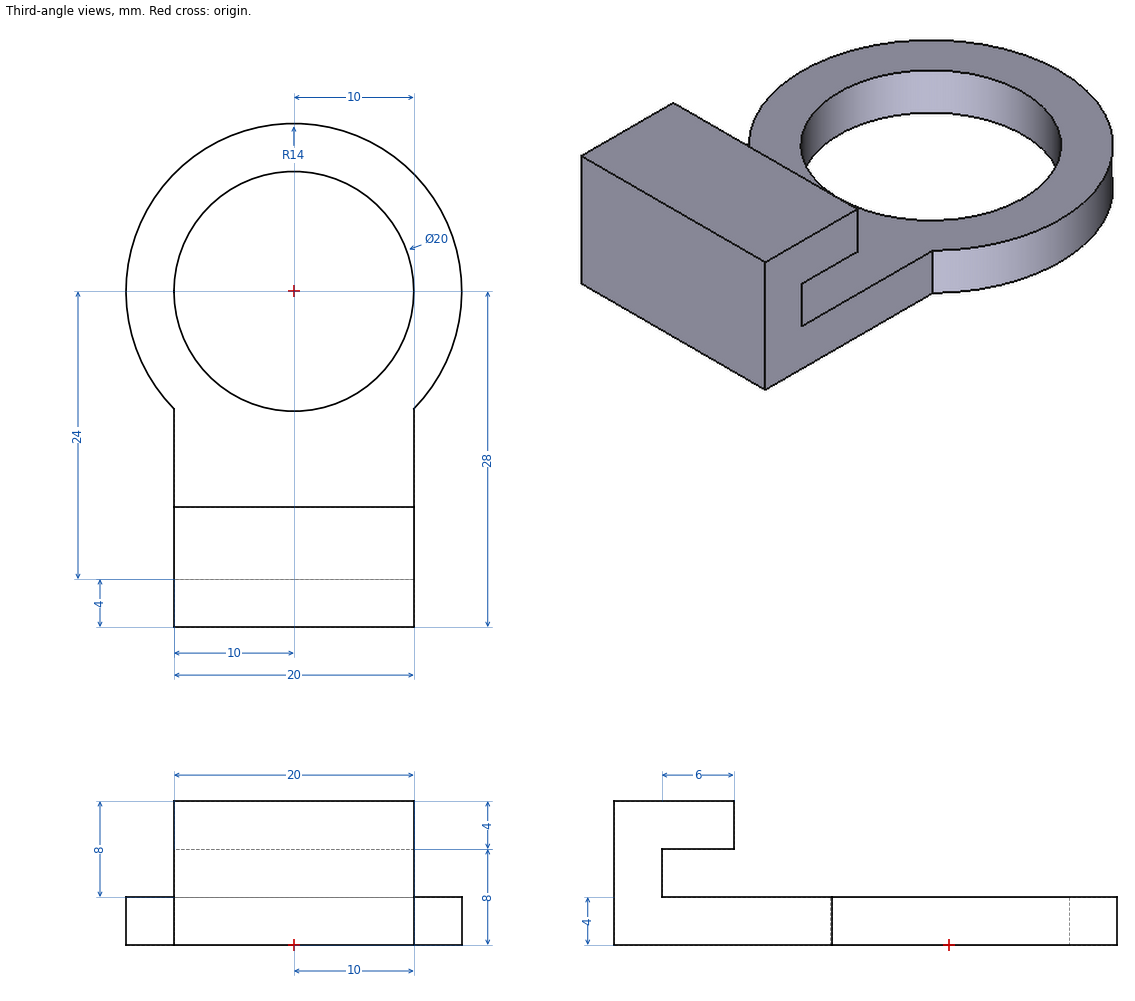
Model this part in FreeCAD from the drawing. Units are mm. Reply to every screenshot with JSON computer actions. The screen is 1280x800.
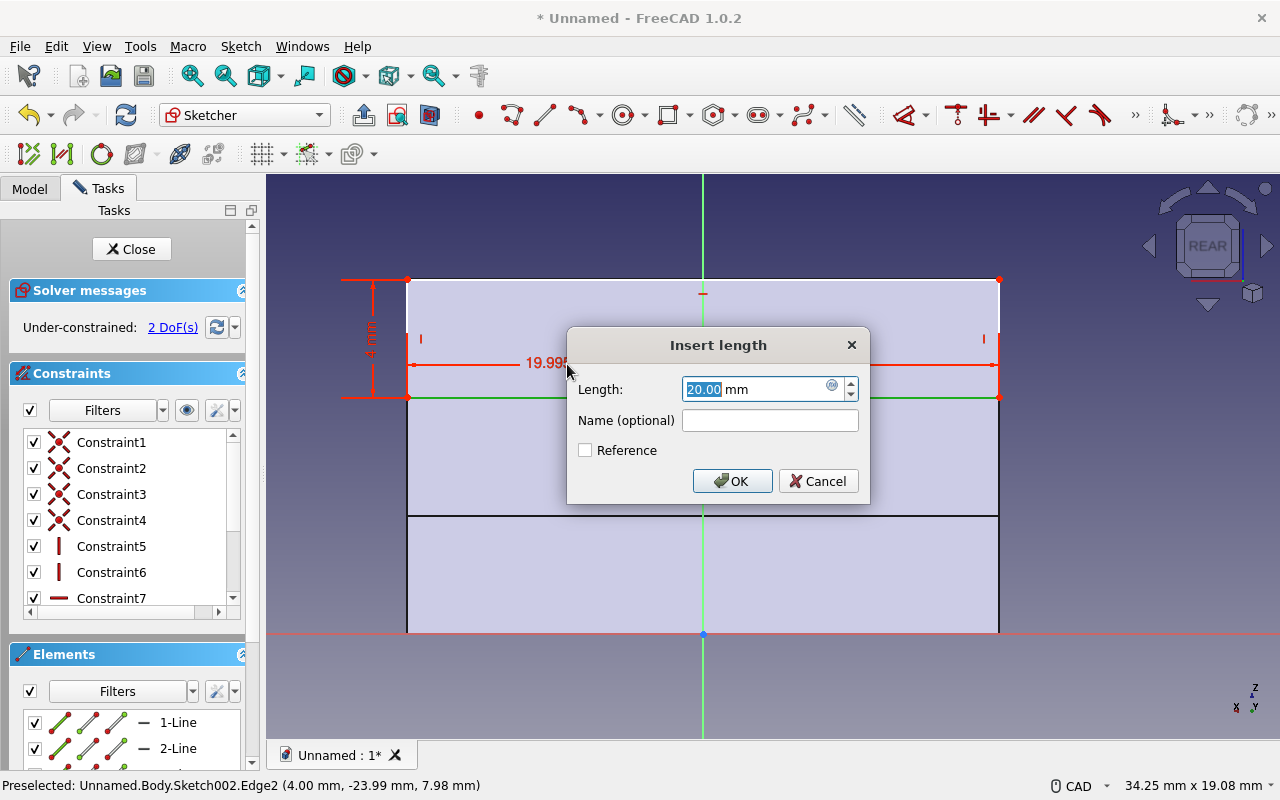
{"action": "type", "text": "20"}
{"action": "key", "text": "Return"}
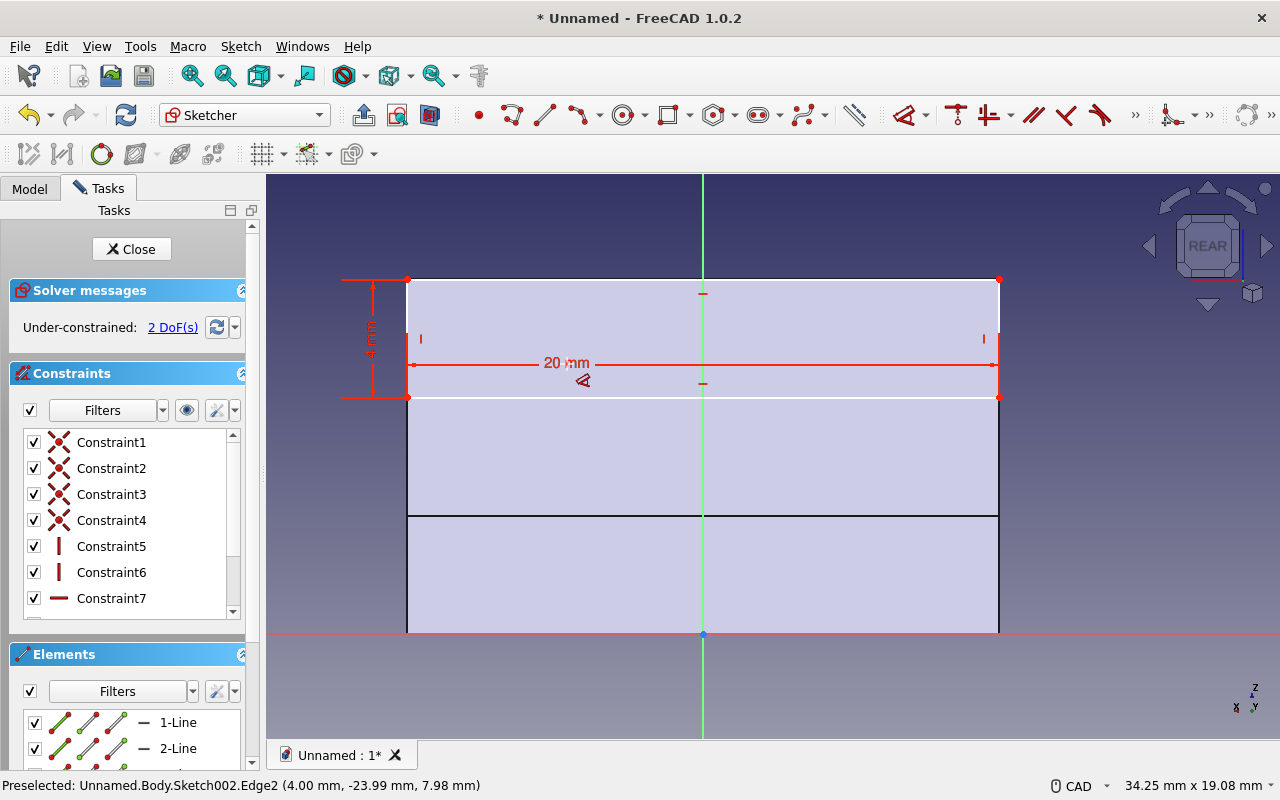
{"action": "left_click", "coordinate": [407, 398]}
{"action": "left_click", "coordinate": [373, 516]}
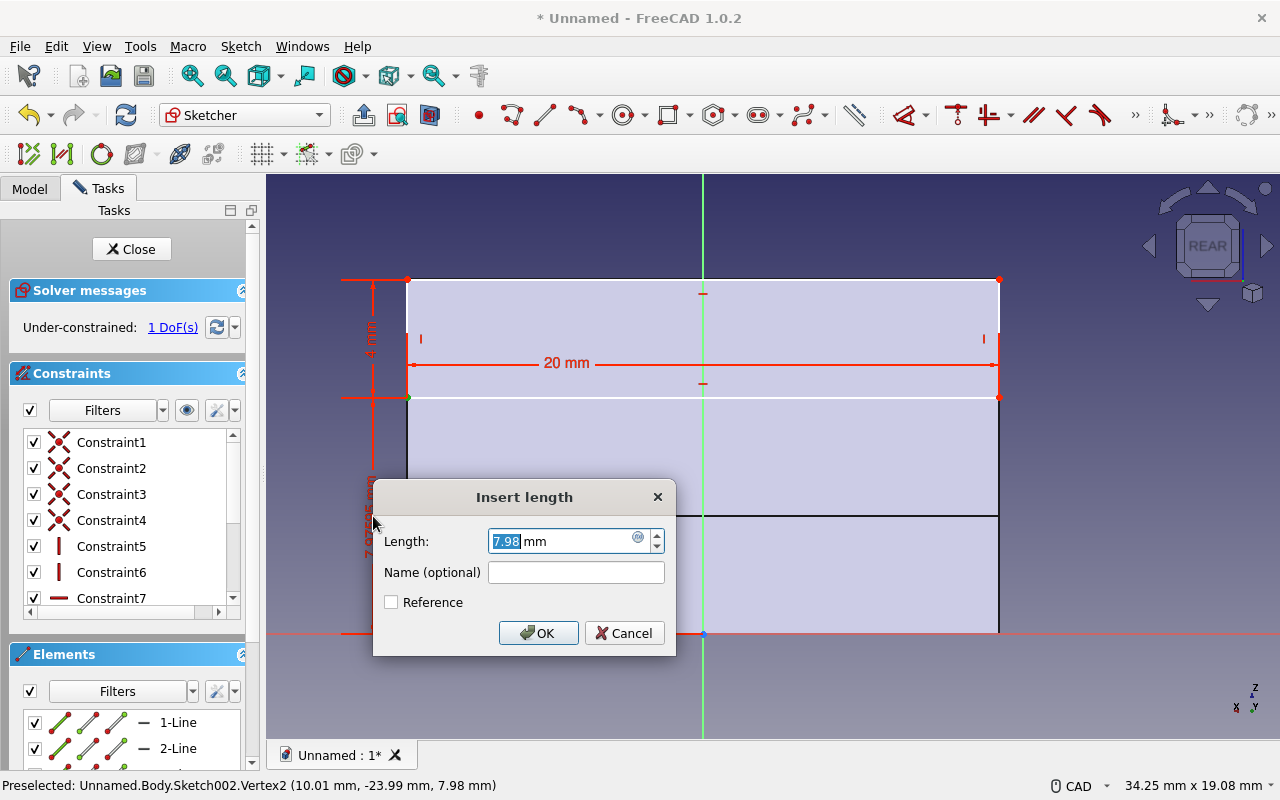
{"action": "type", "text": "8"}
{"action": "key", "text": "Return"}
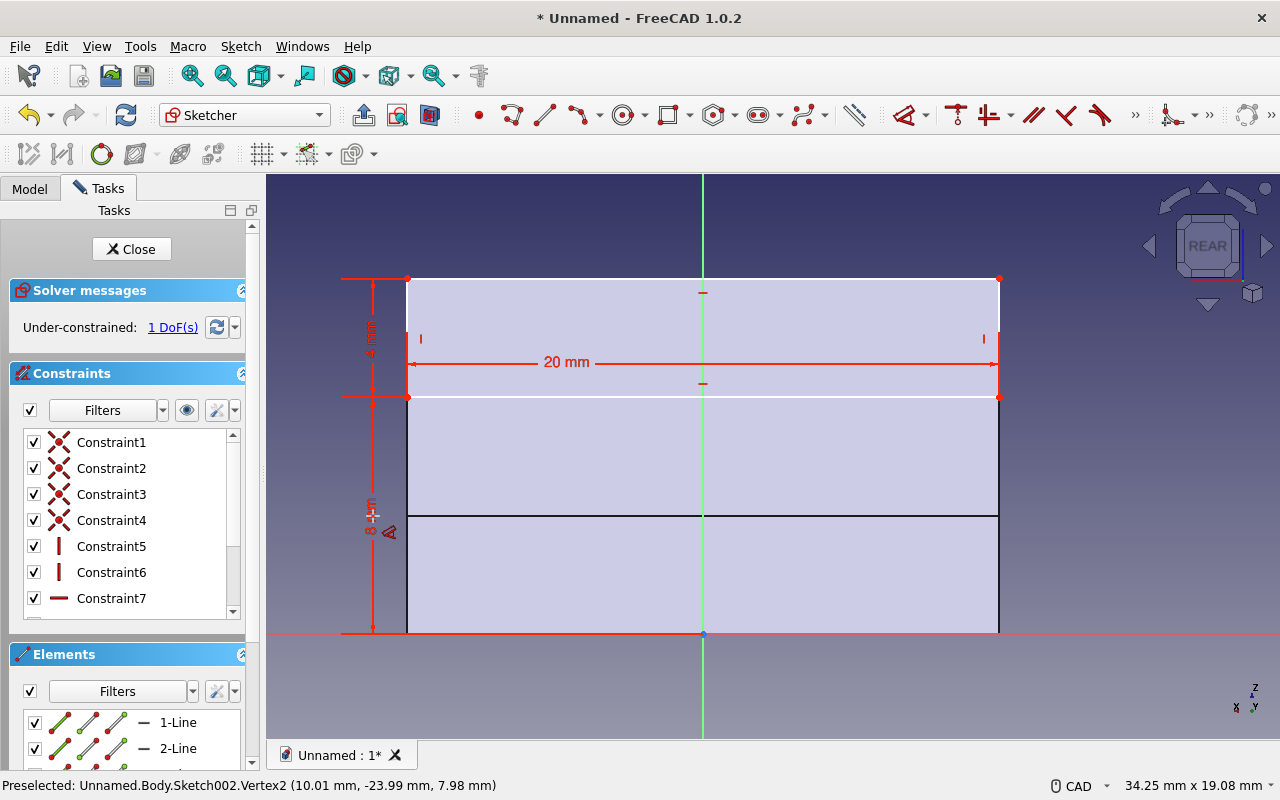
{"action": "left_click", "coordinate": [407, 279]}
{"action": "left_click", "coordinate": [555, 668]}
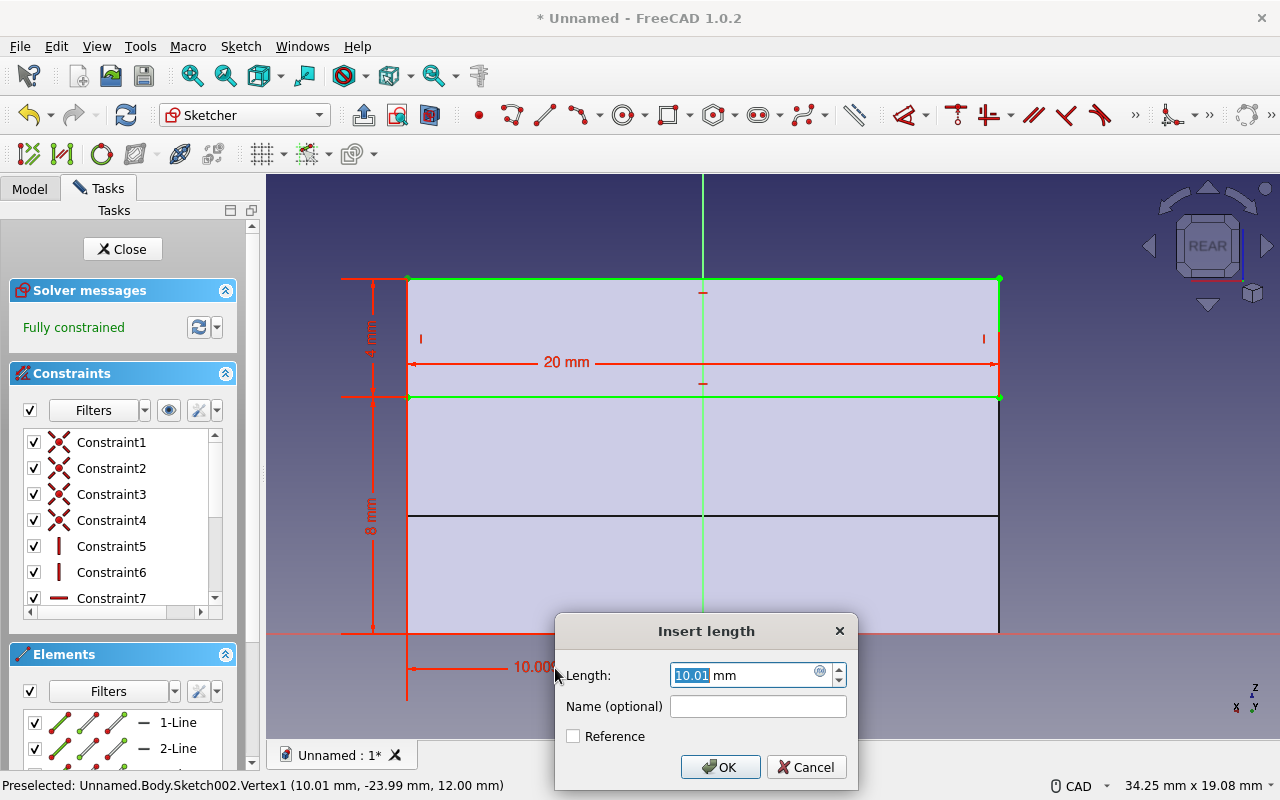
{"action": "type", "text": "10"}
{"action": "key", "text": "Return"}
{"action": "key", "text": "Escape"}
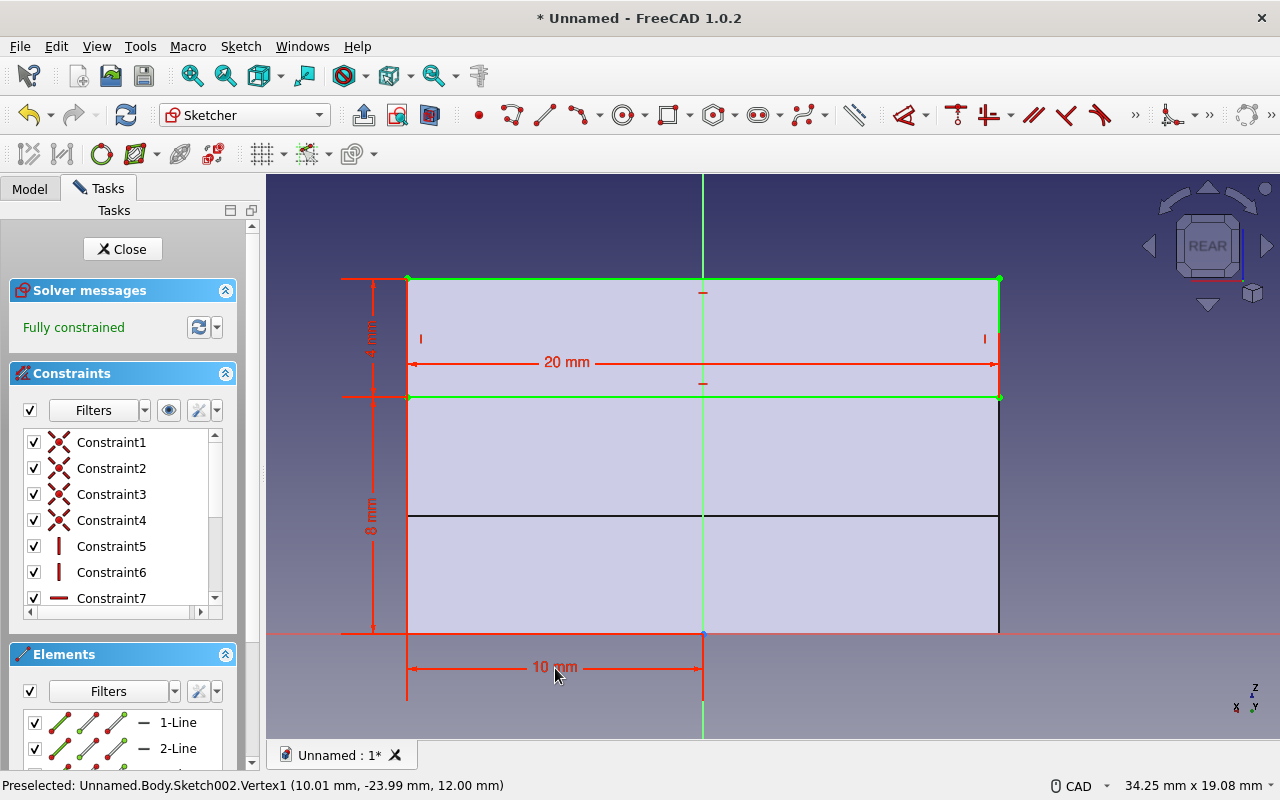
{"action": "left_click", "coordinate": [123, 249]}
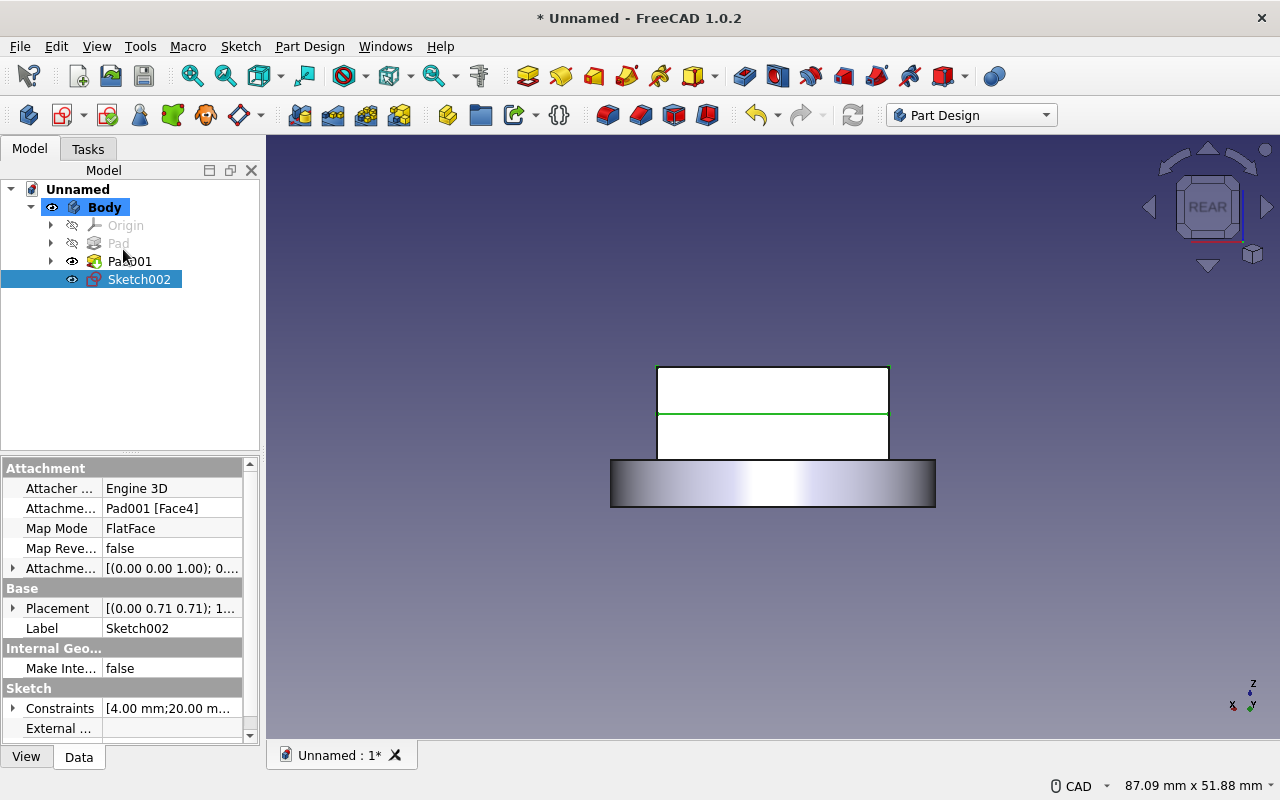
{"action": "left_click", "coordinate": [528, 76]}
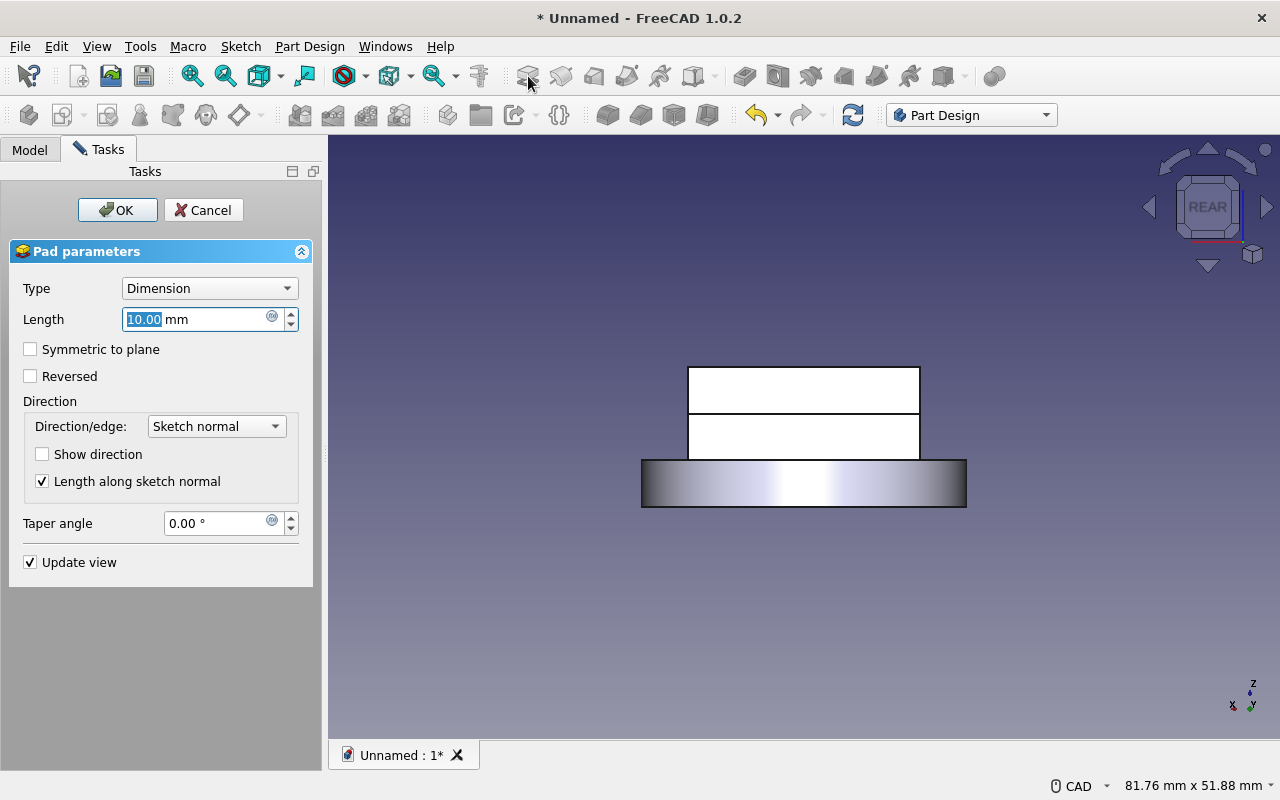
{"action": "type", "text": "6"}
{"action": "key", "text": "Tab"}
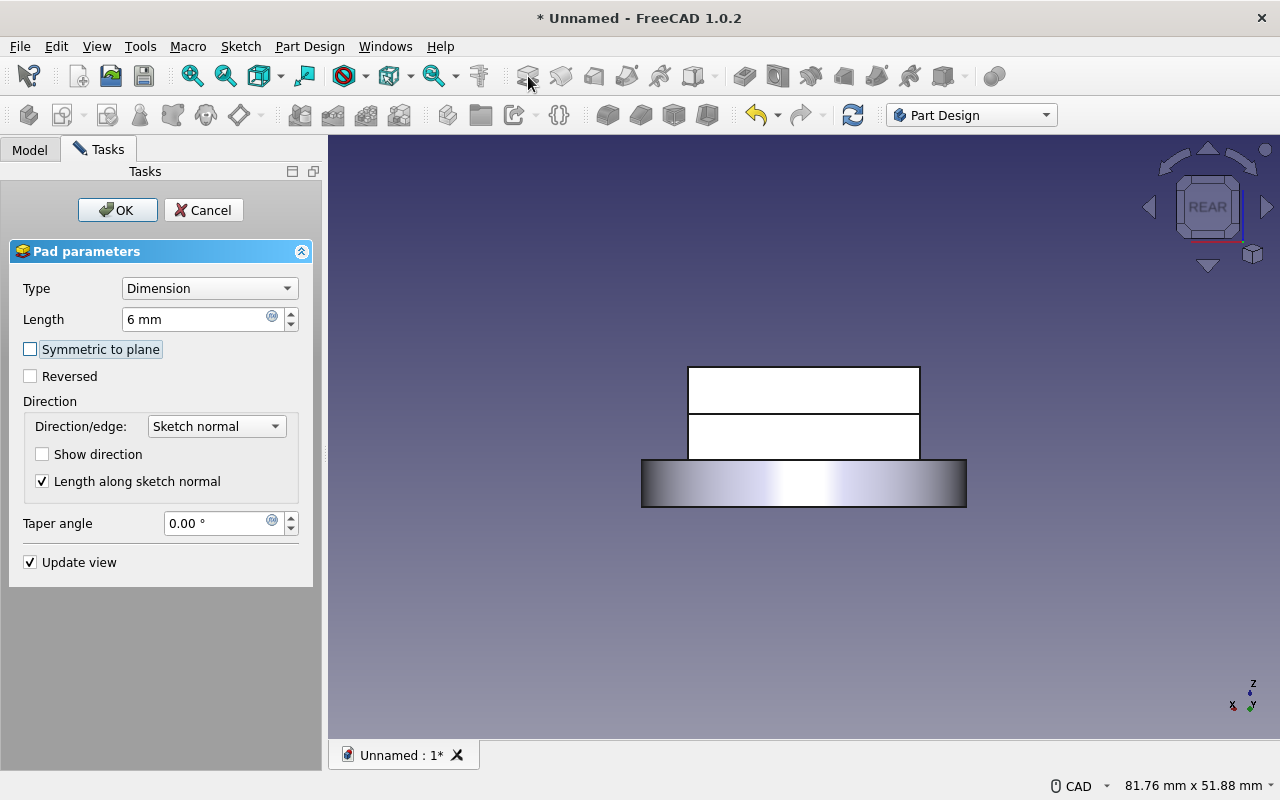
{"action": "left_click", "coordinate": [118, 210]}